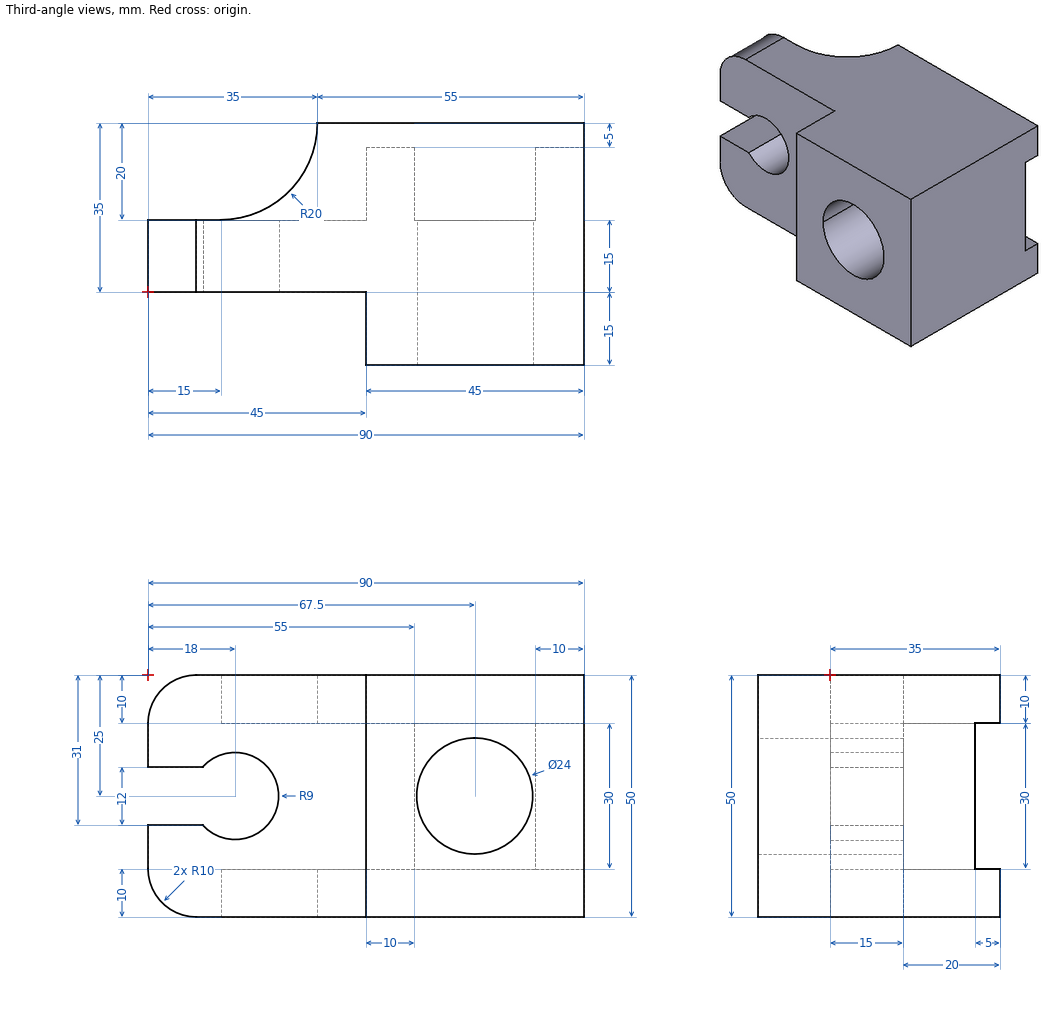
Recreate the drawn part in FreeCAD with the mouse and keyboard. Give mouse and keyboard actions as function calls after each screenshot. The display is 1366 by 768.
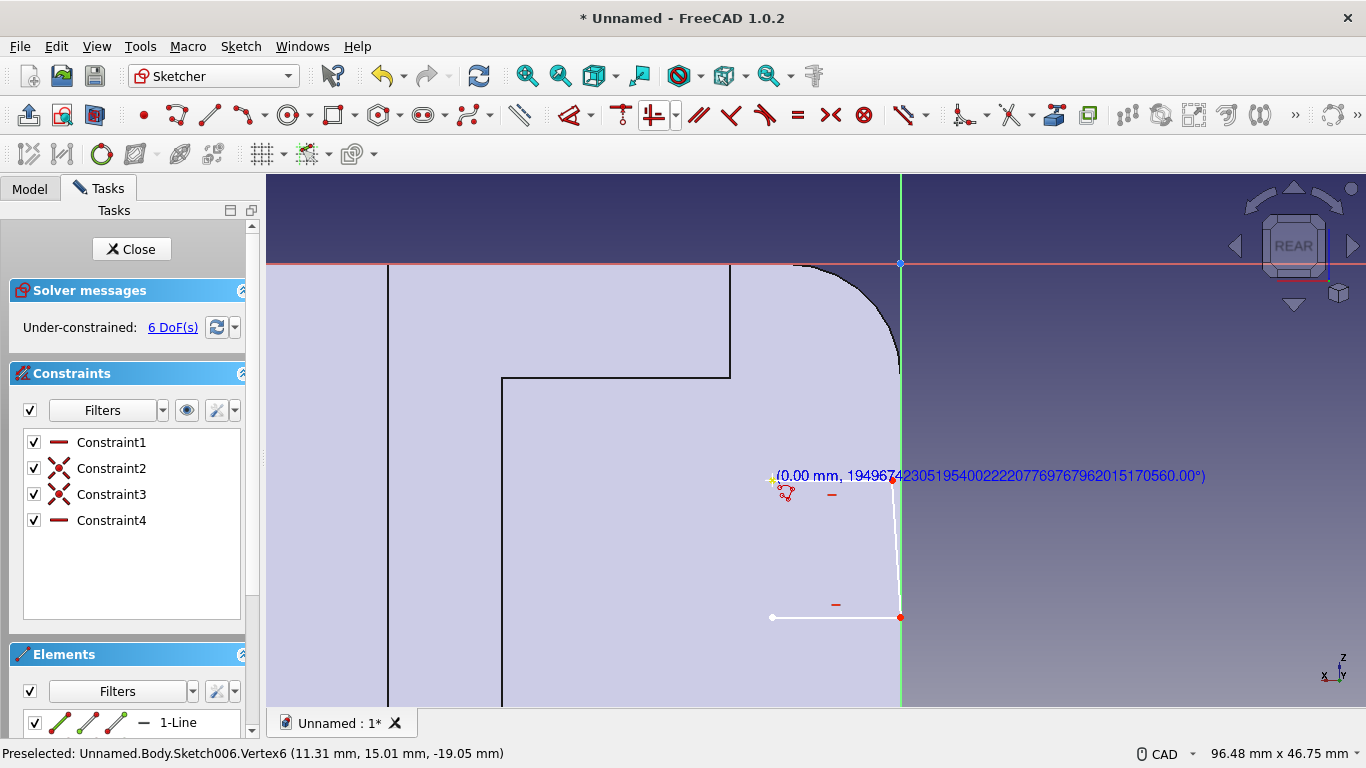
click(242, 116)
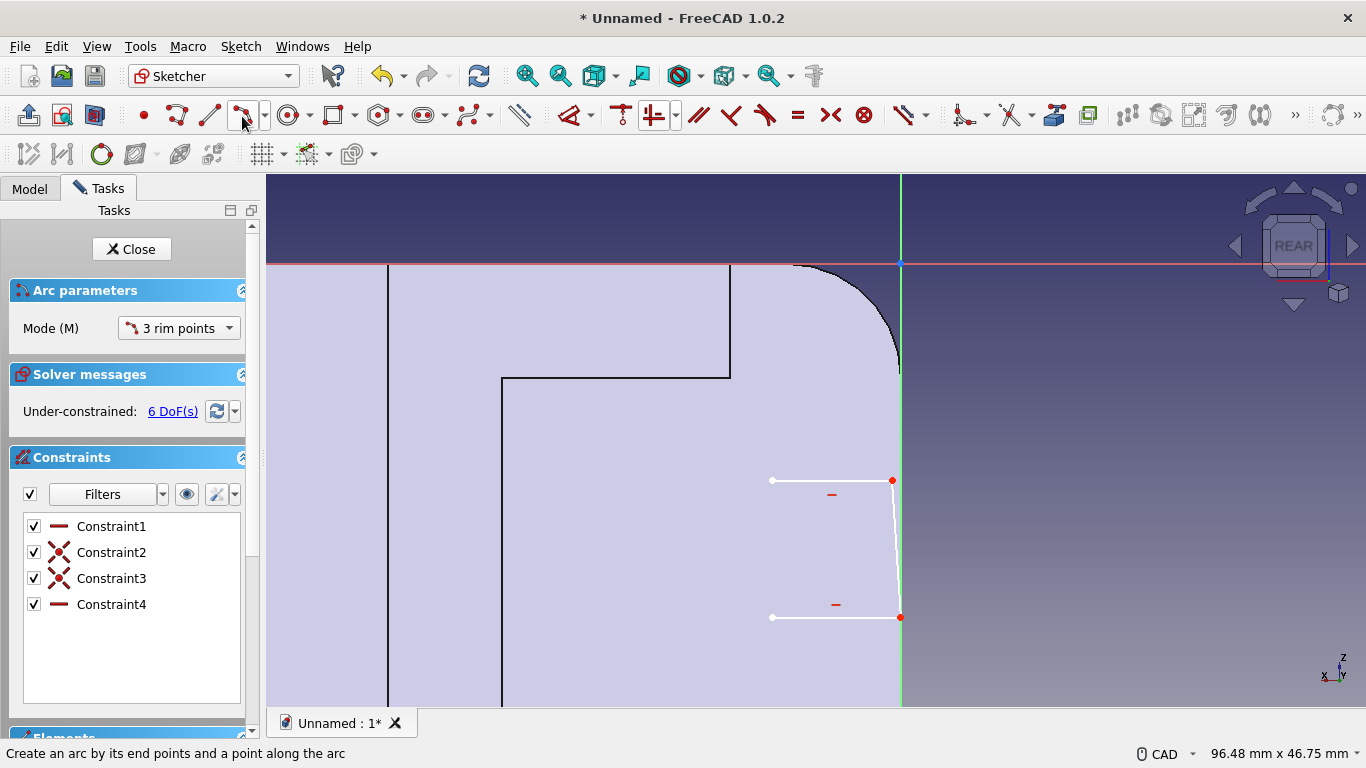
click(772, 481)
click(772, 618)
click(593, 549)
key(Escape)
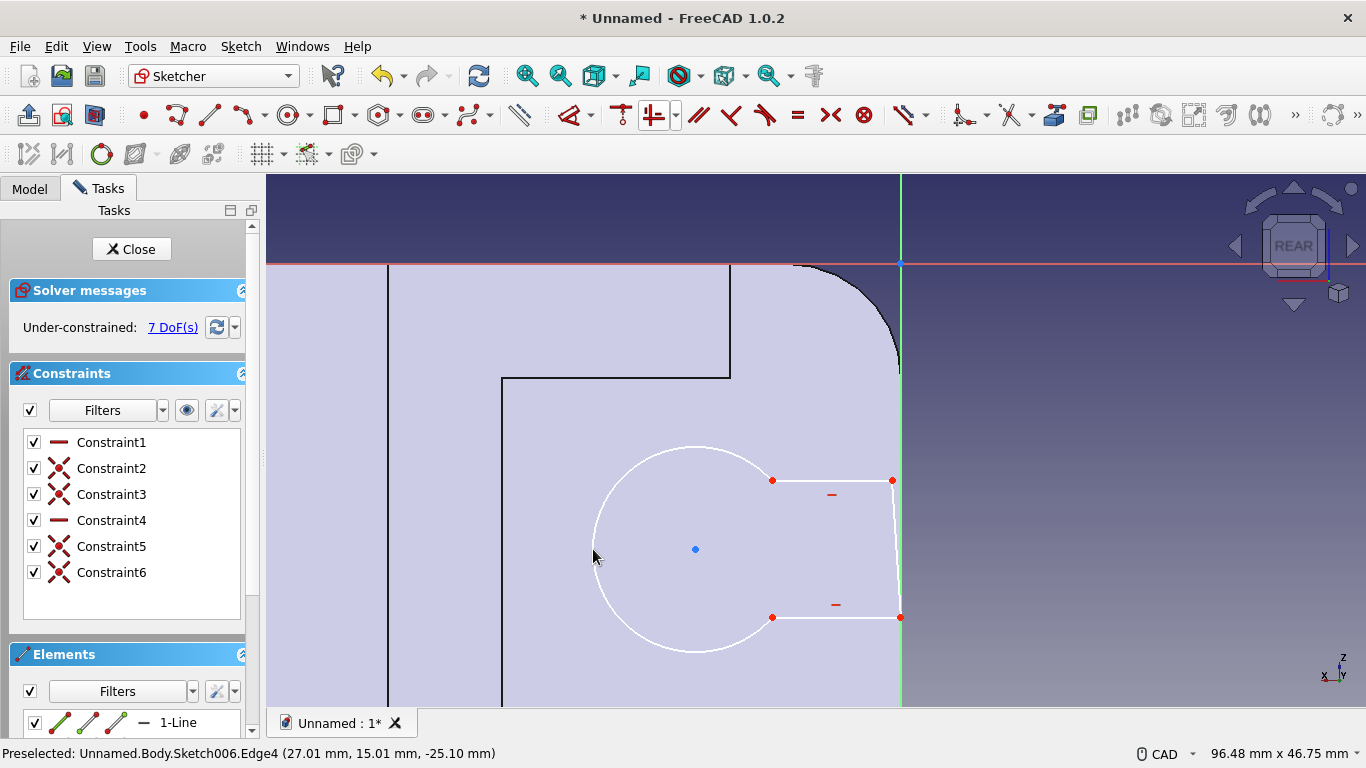
click(898, 577)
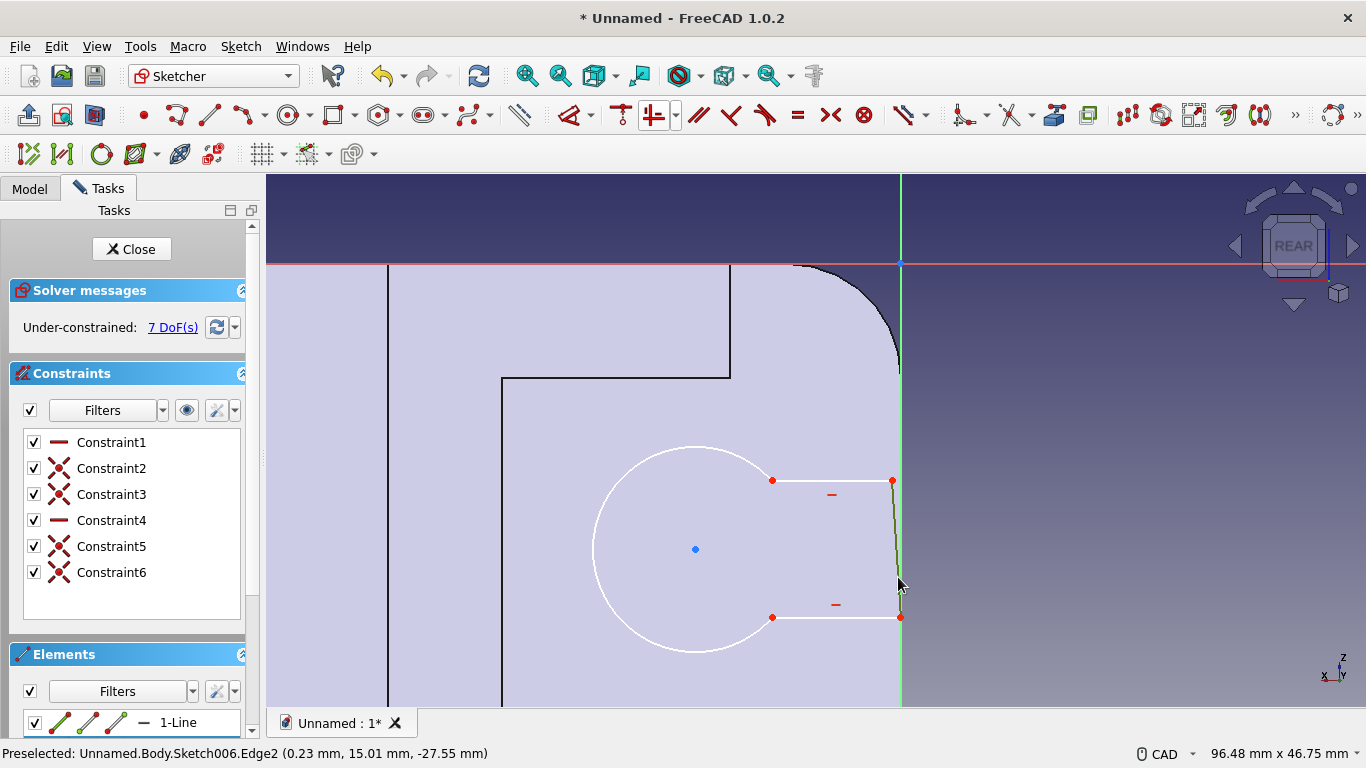
key(v)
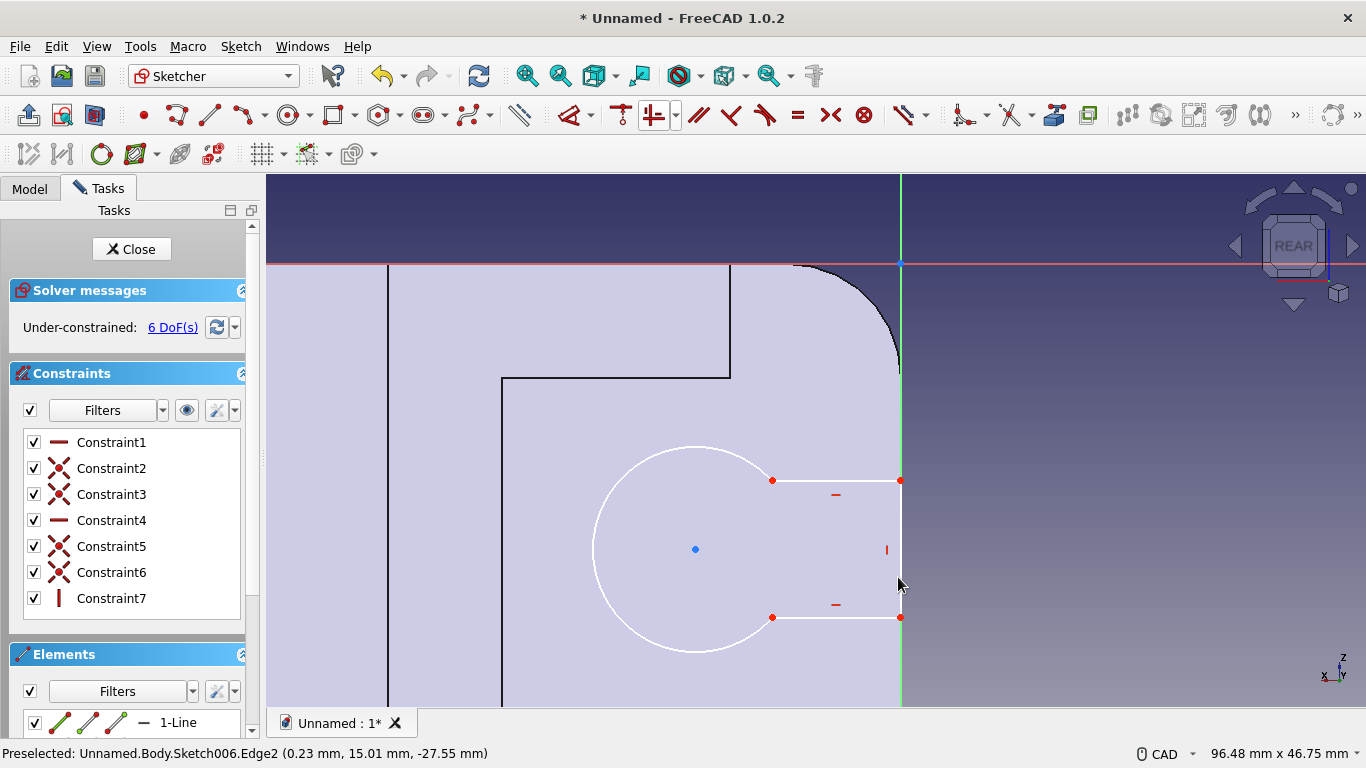
click(568, 116)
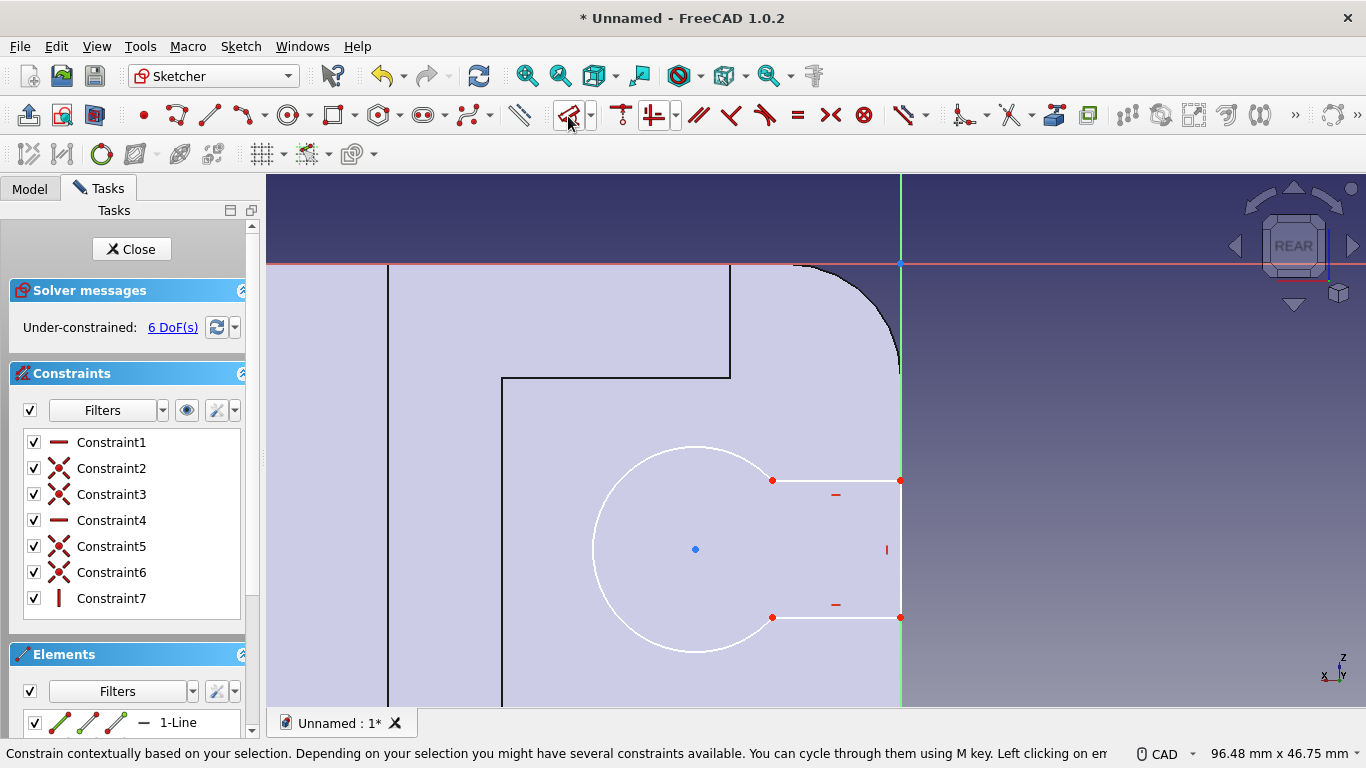
click(637, 465)
click(619, 439)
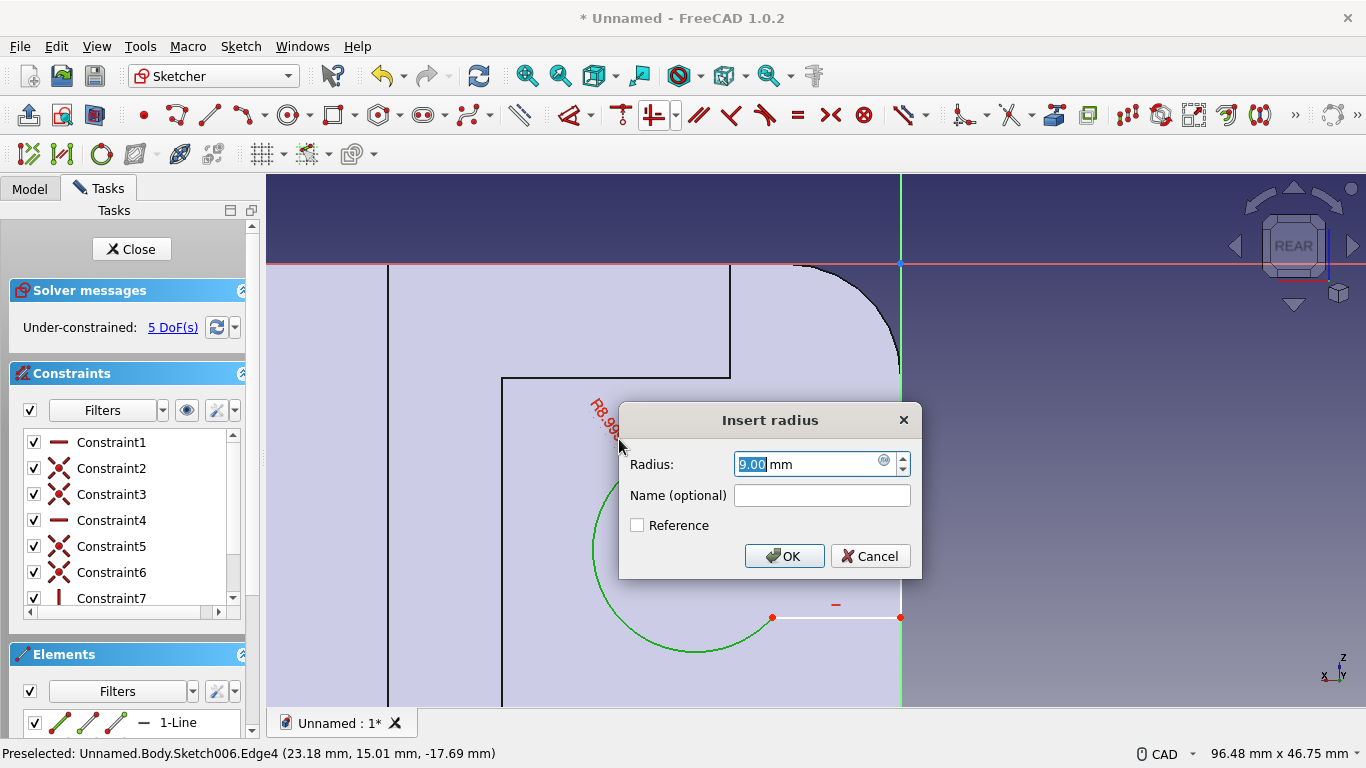
text(9)
key(Return)
key(Escape)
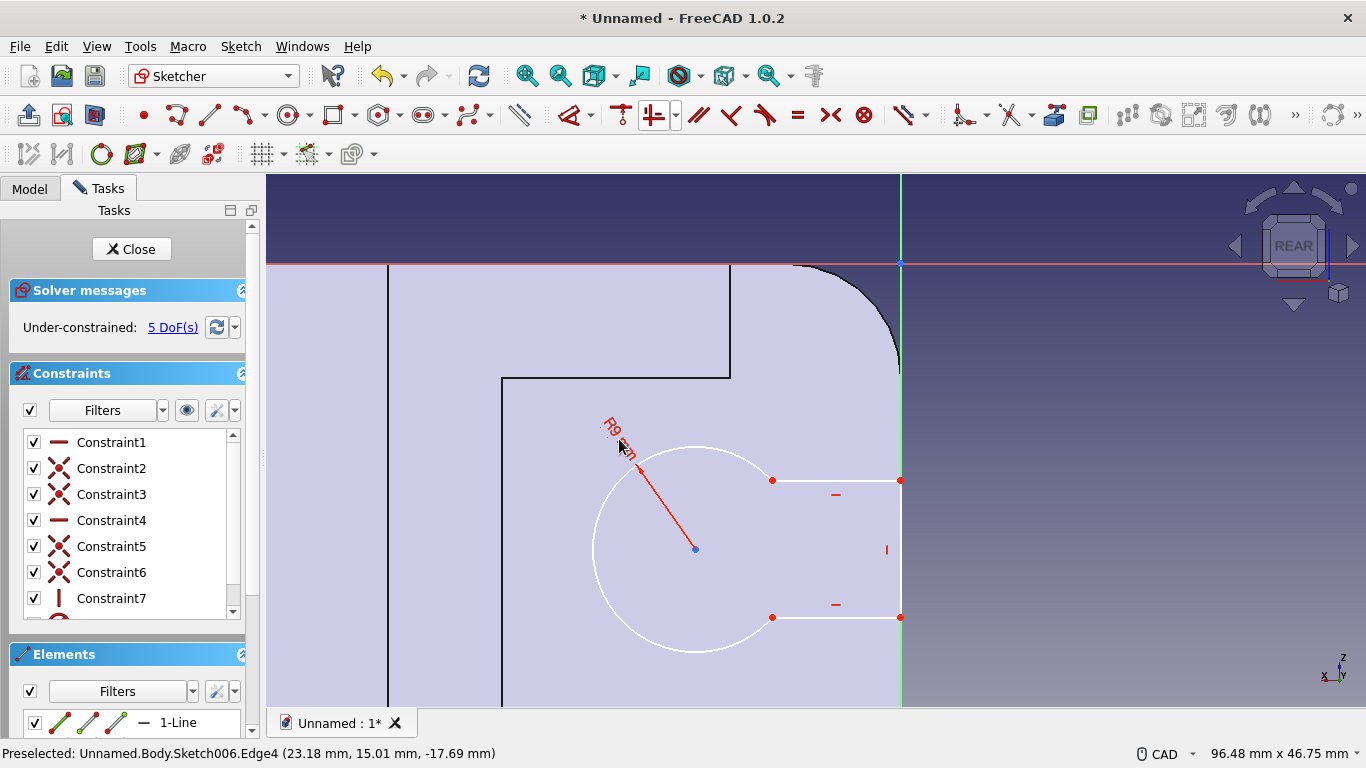
click(901, 618)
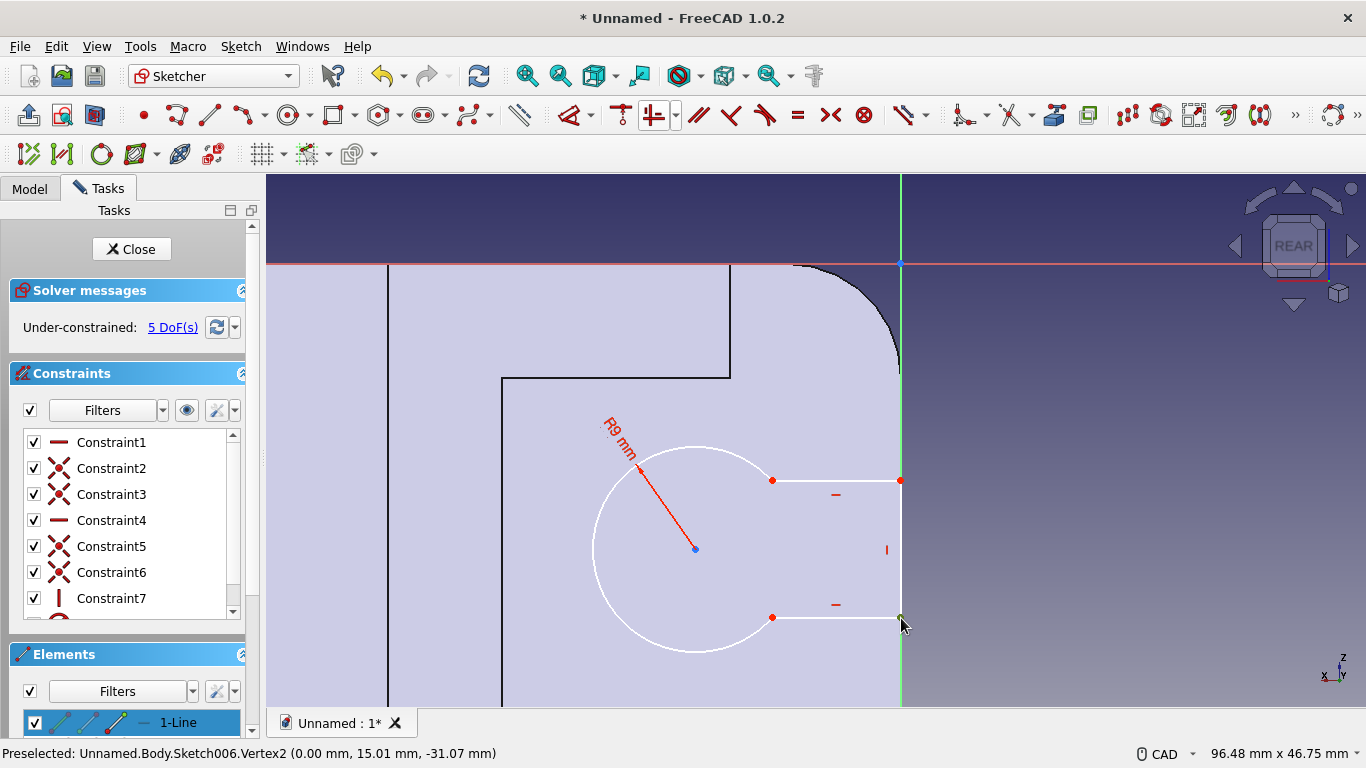
click(901, 440)